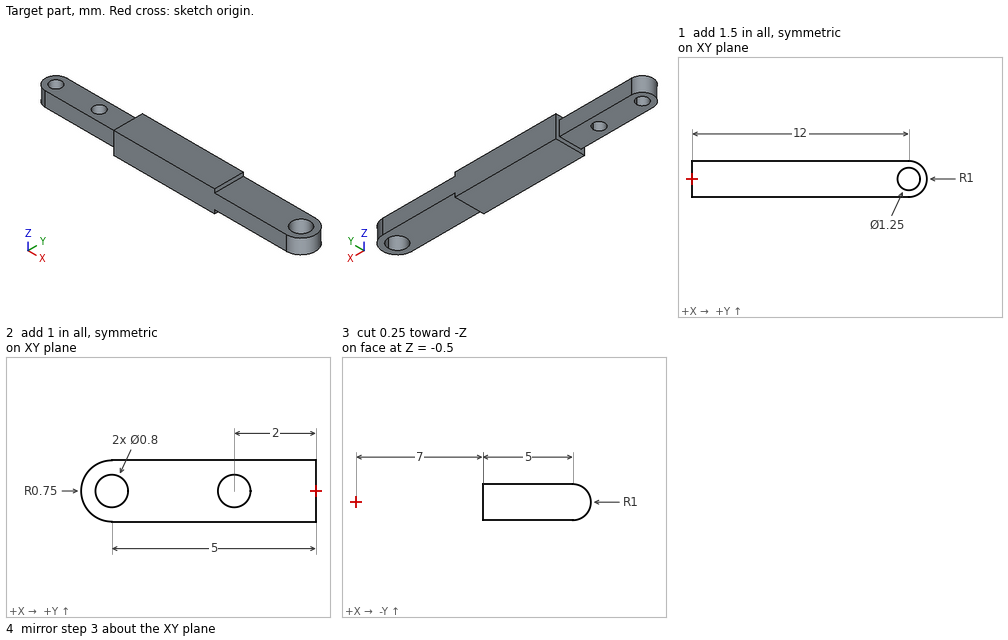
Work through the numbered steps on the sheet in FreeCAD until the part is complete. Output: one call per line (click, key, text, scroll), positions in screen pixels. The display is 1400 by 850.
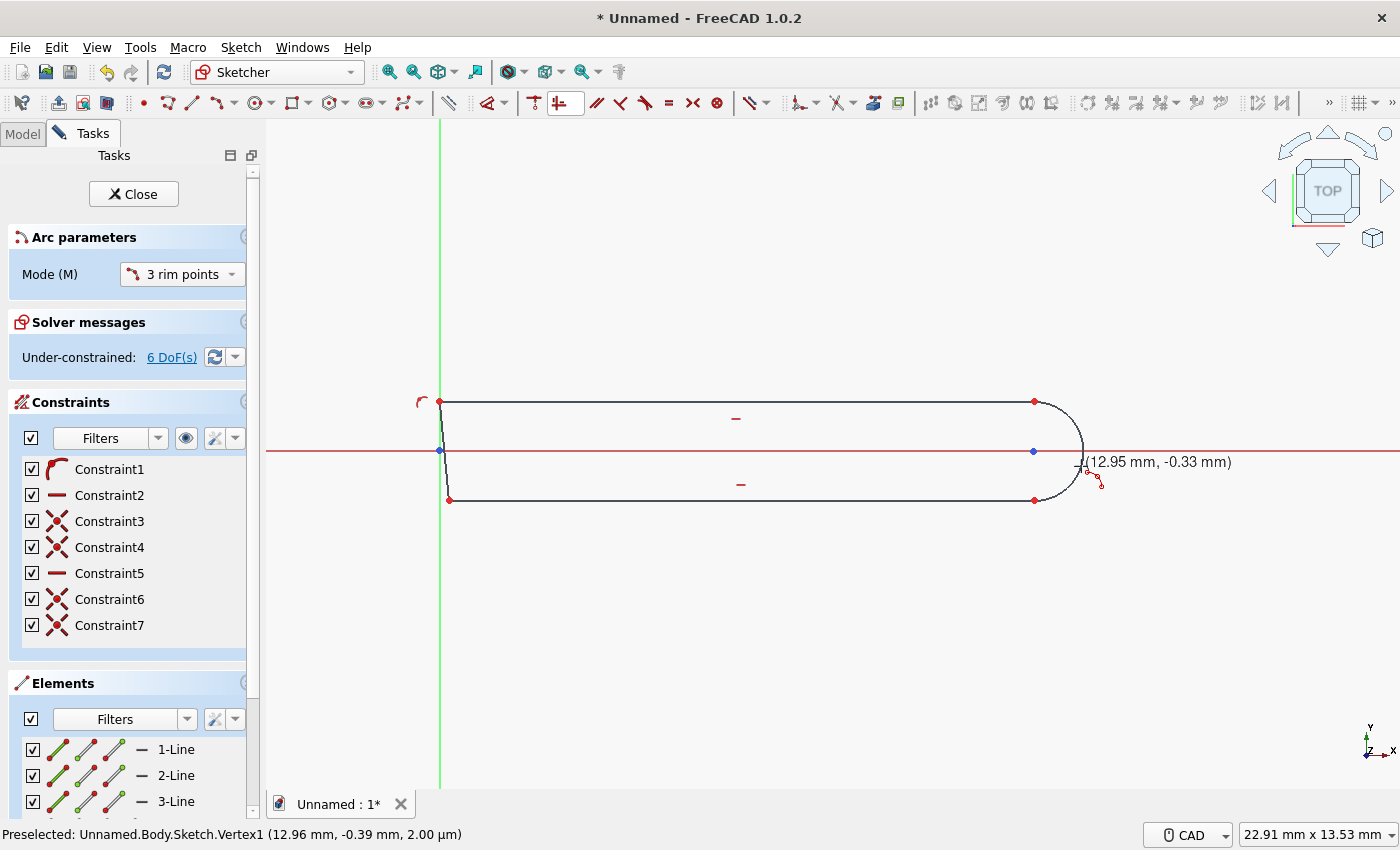
click(256, 104)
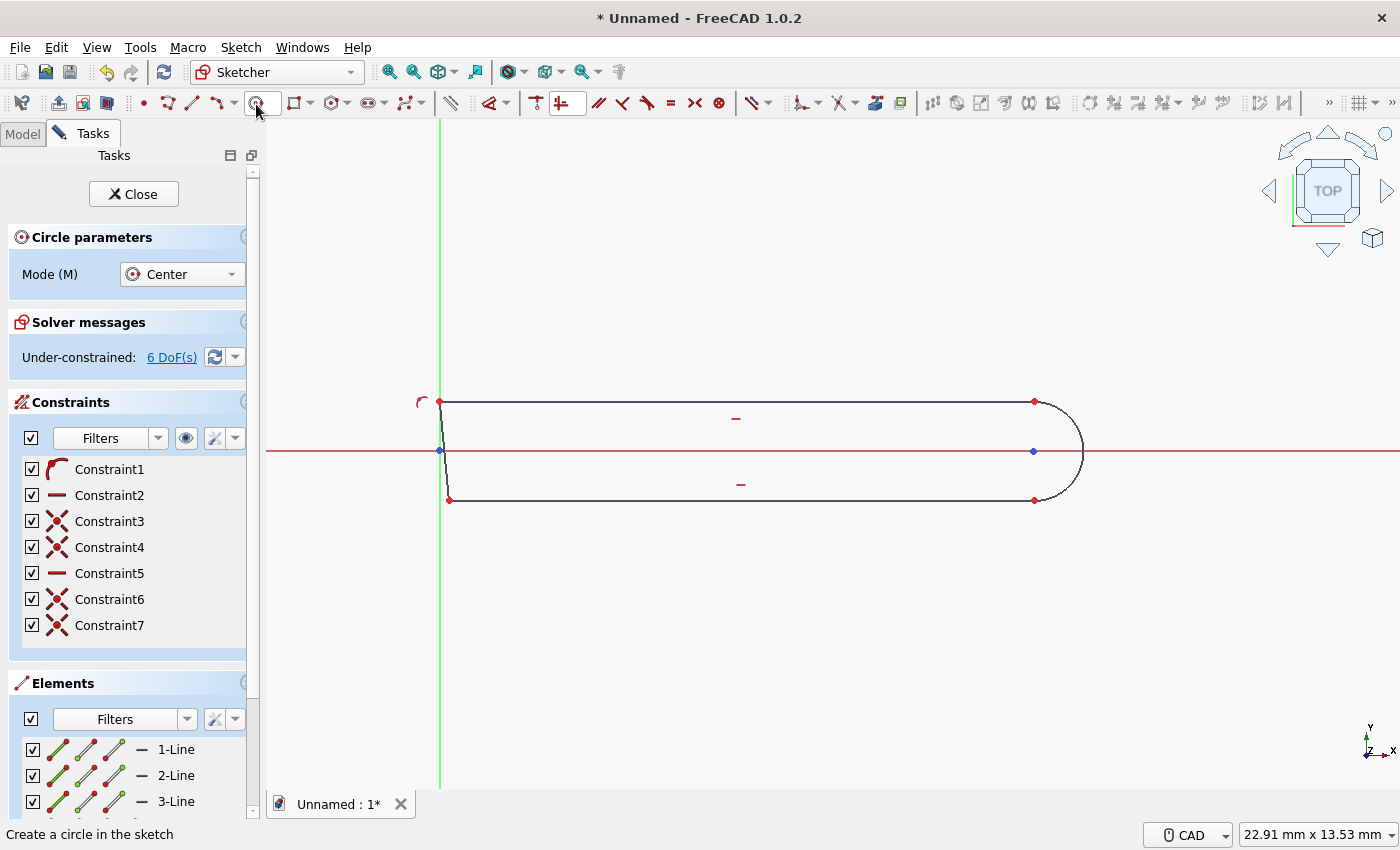
click(1034, 451)
move(1056, 429)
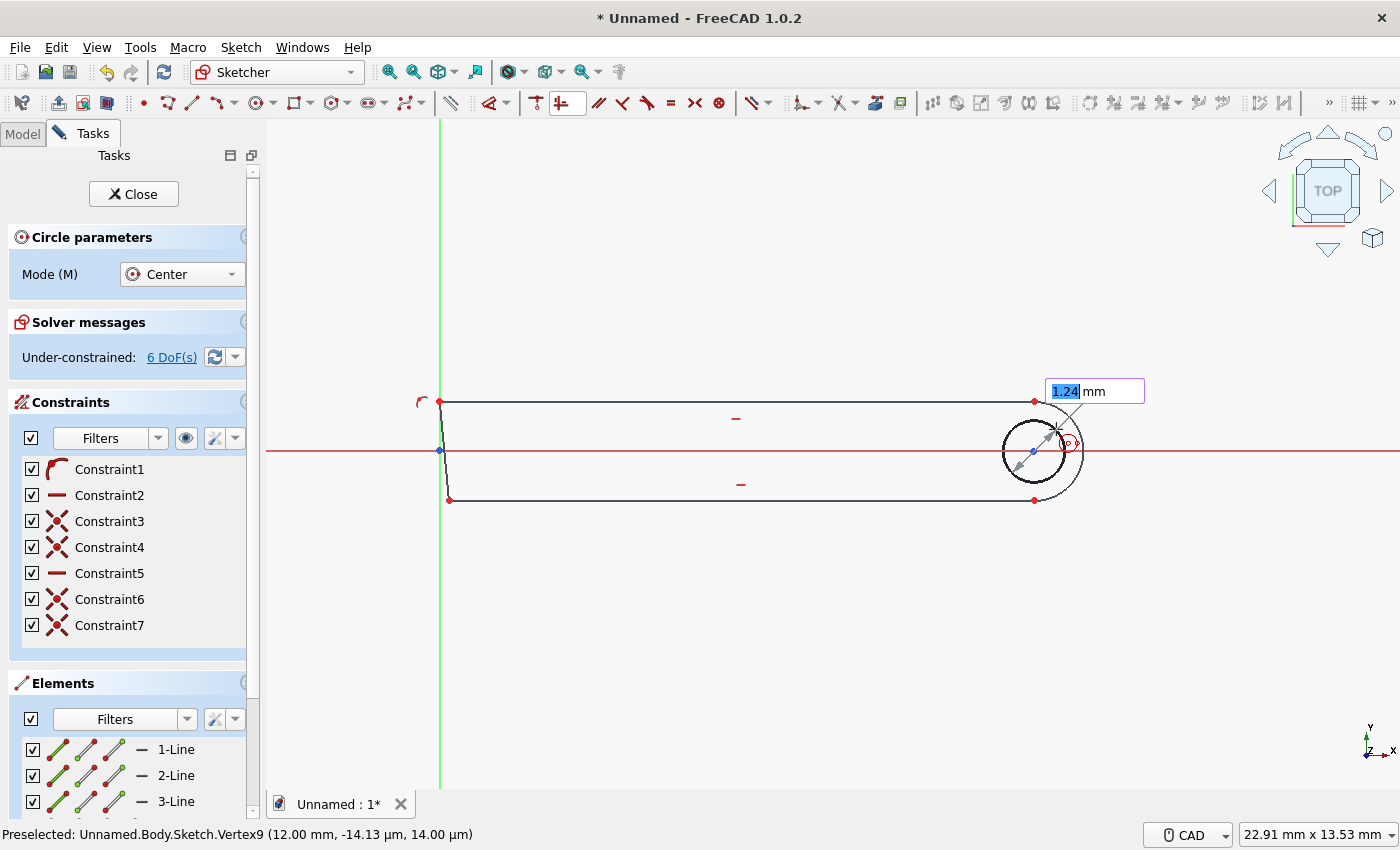
text(1.25)
key(Return)
key(Escape)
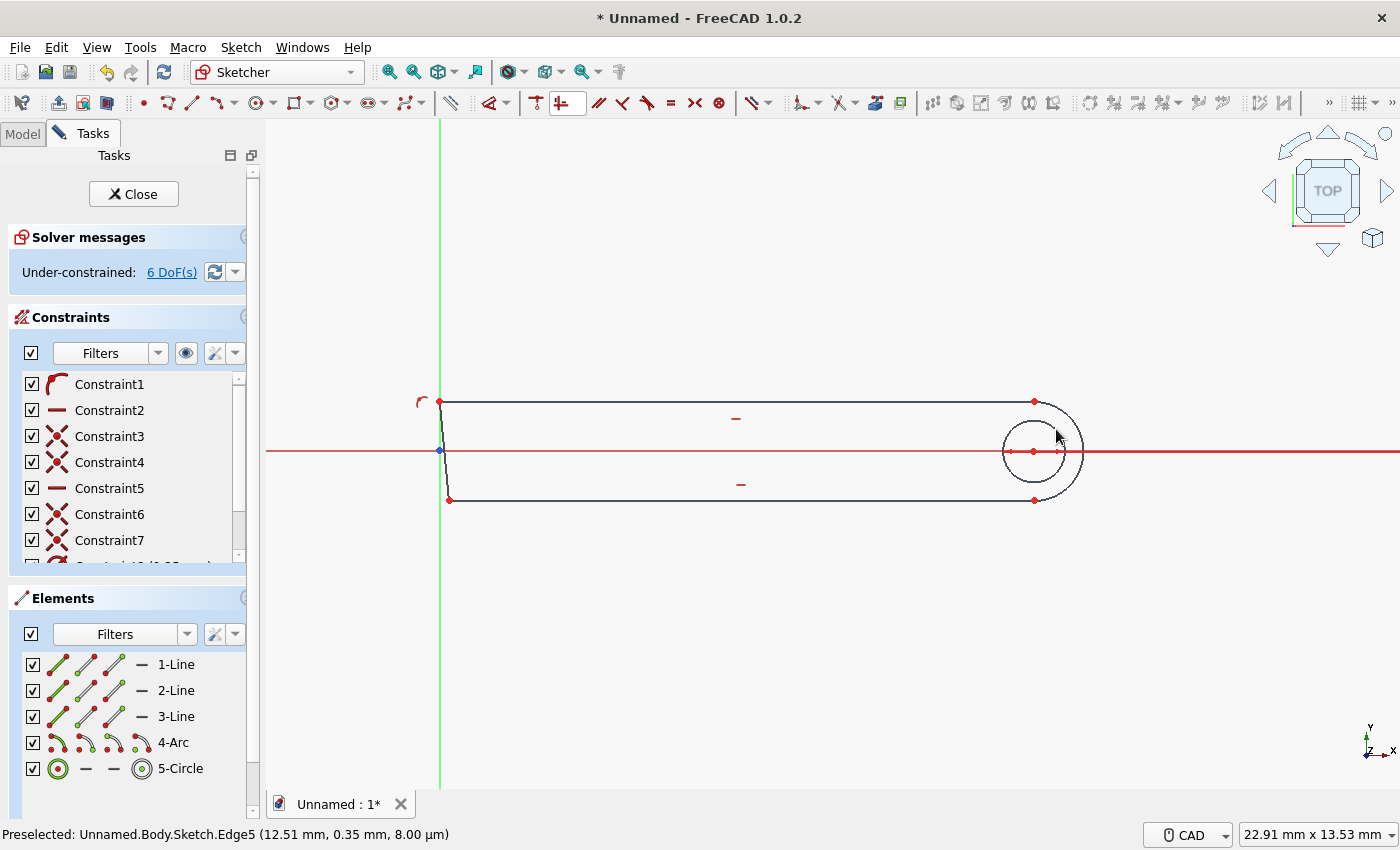
click(856, 402)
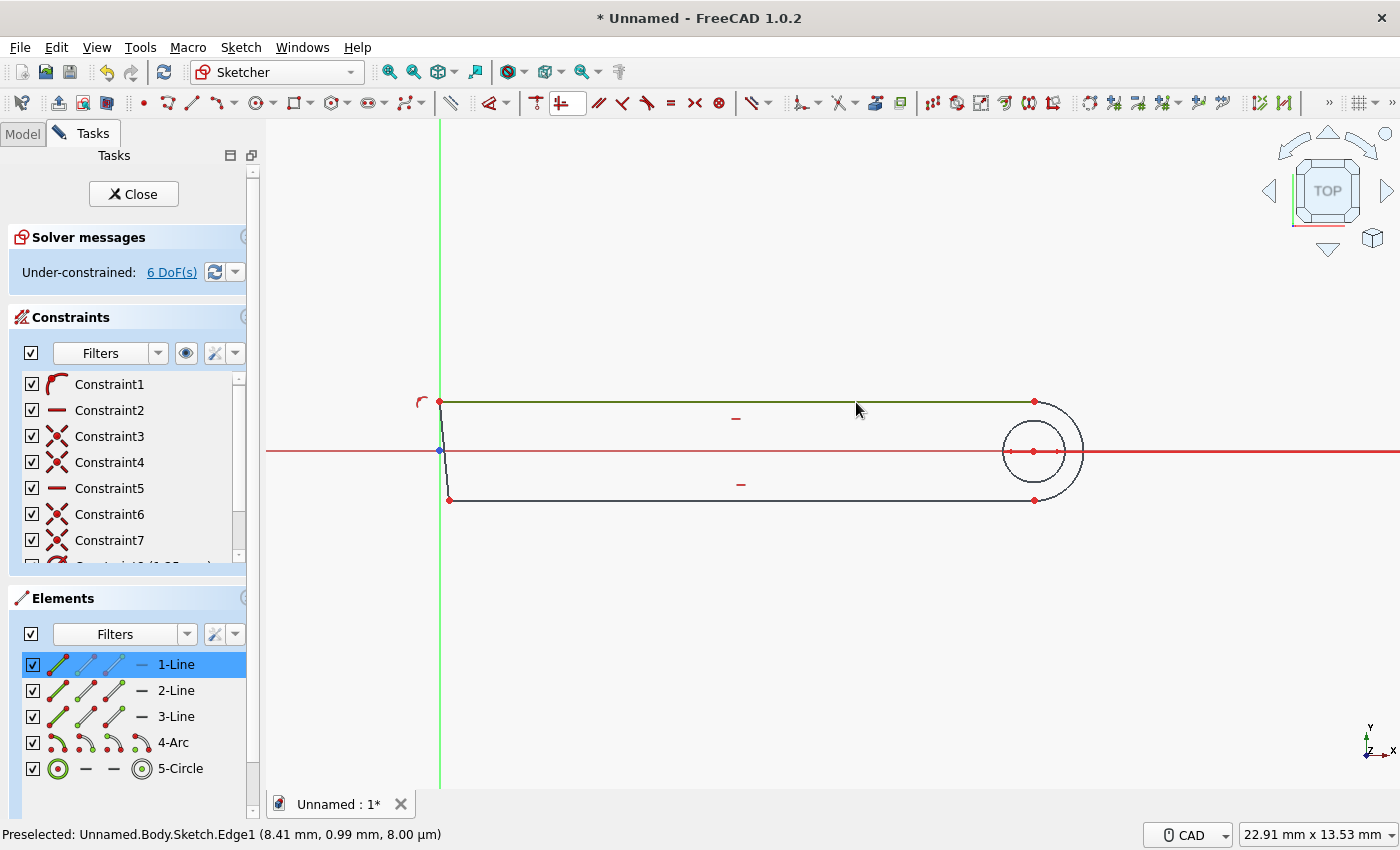
click(1074, 481)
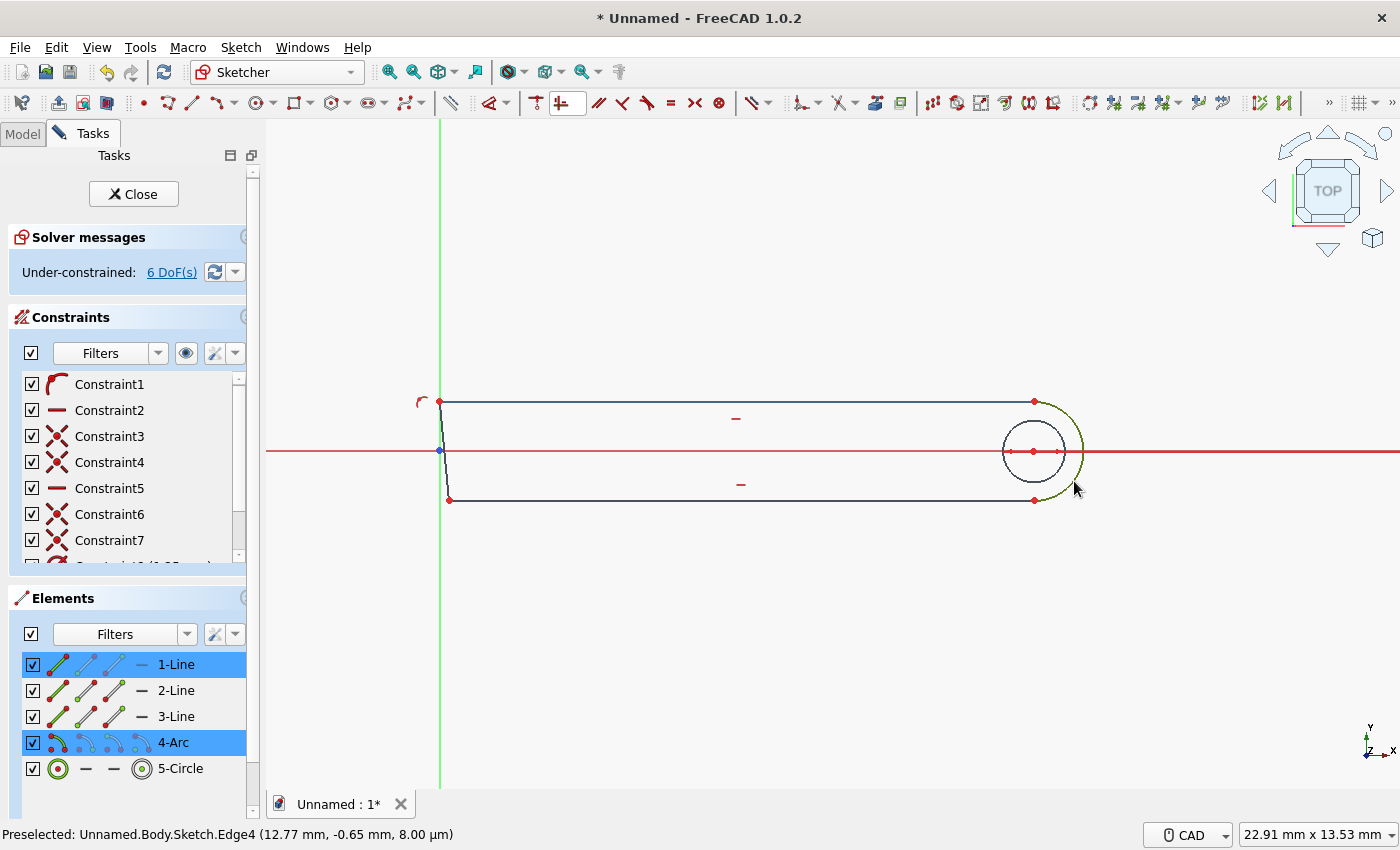
click(648, 104)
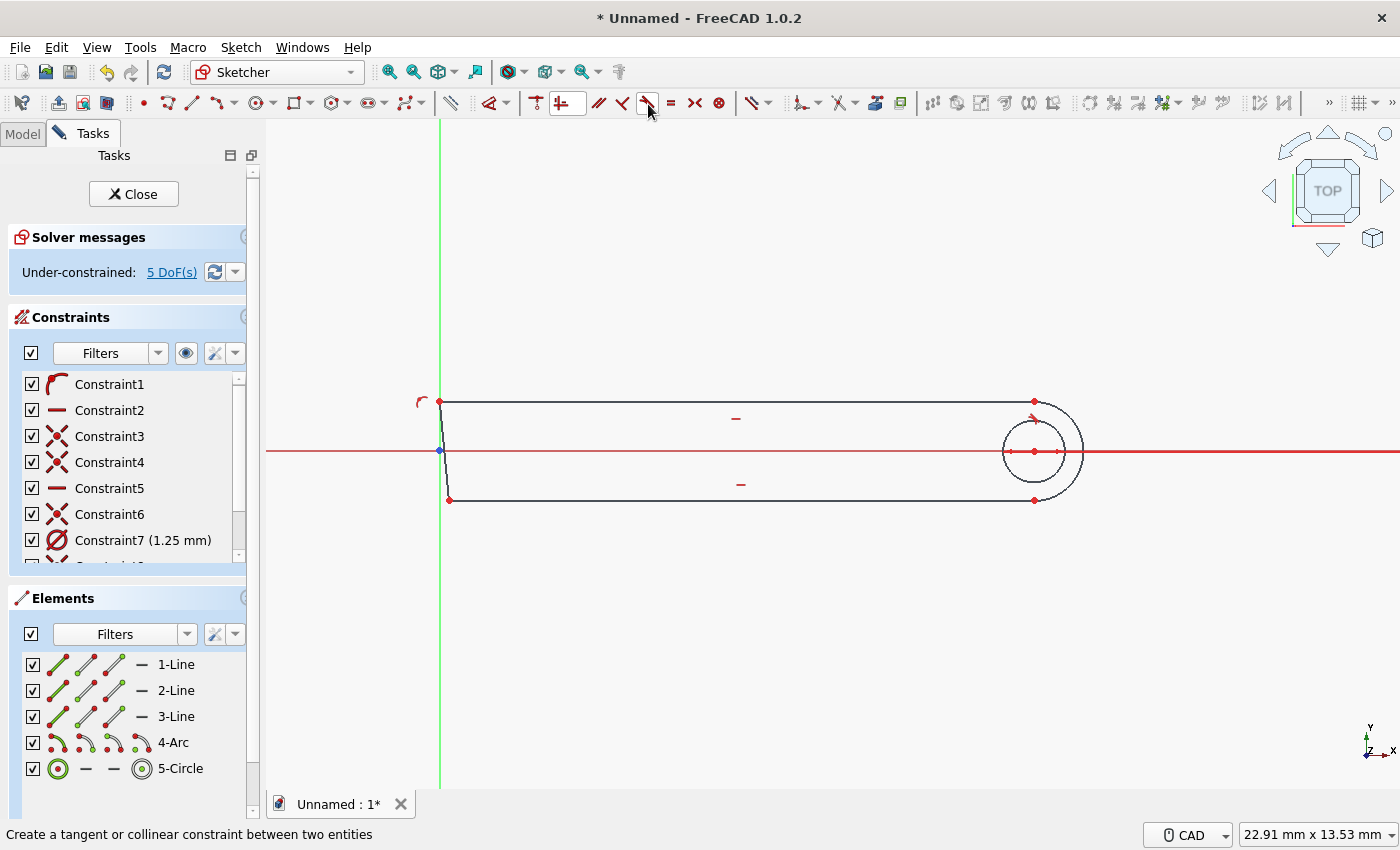
click(625, 501)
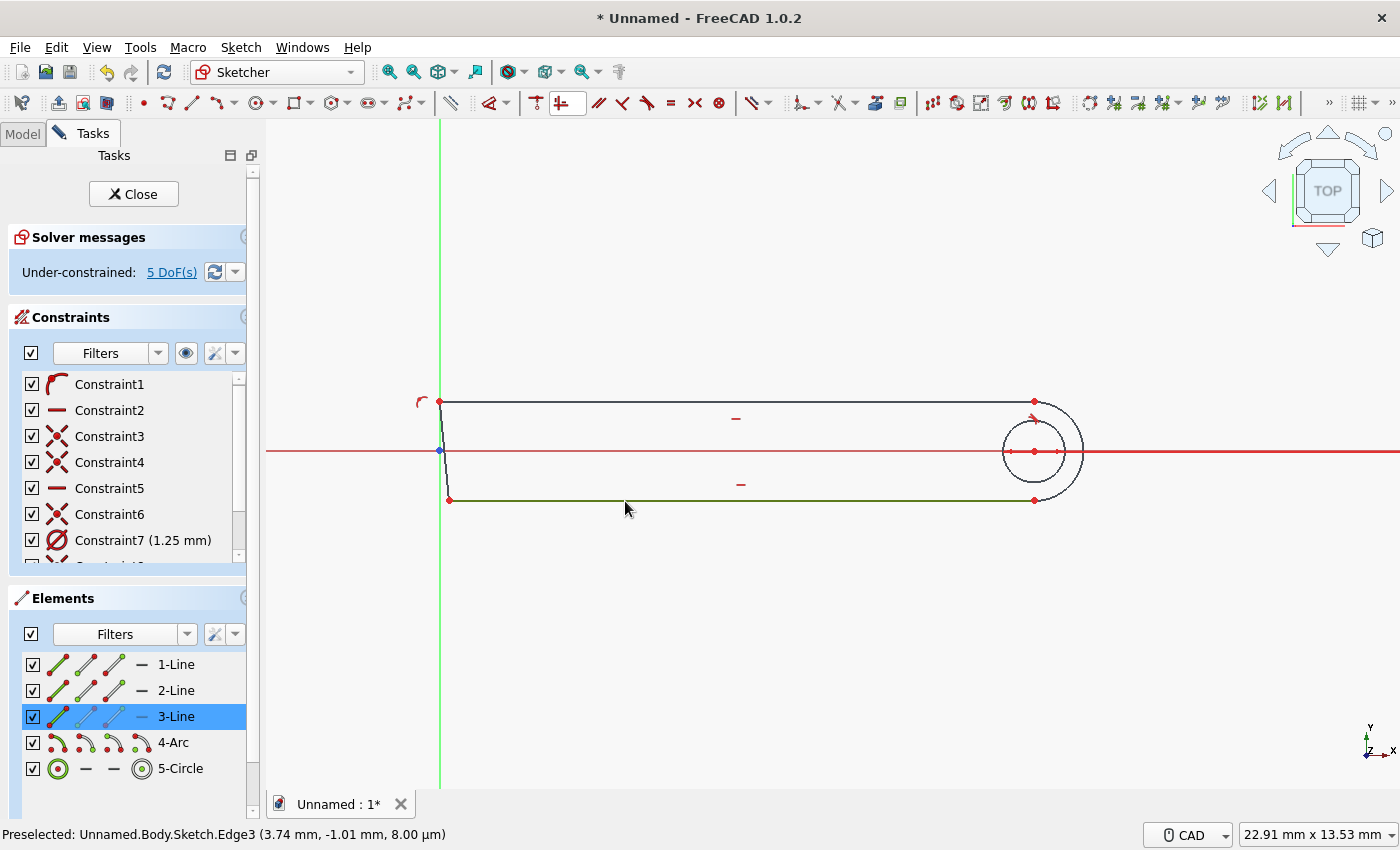
click(1074, 481)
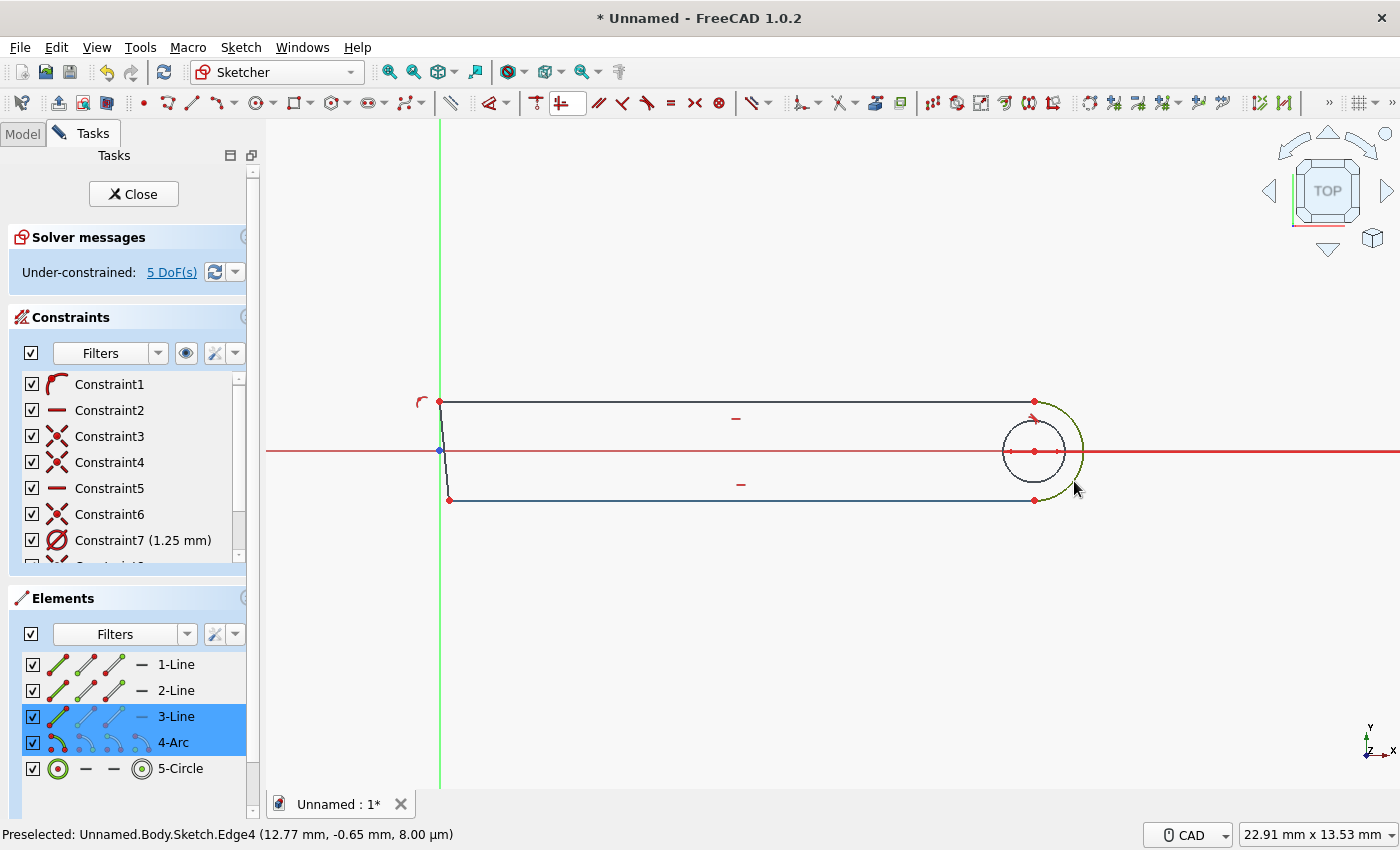
key(t)